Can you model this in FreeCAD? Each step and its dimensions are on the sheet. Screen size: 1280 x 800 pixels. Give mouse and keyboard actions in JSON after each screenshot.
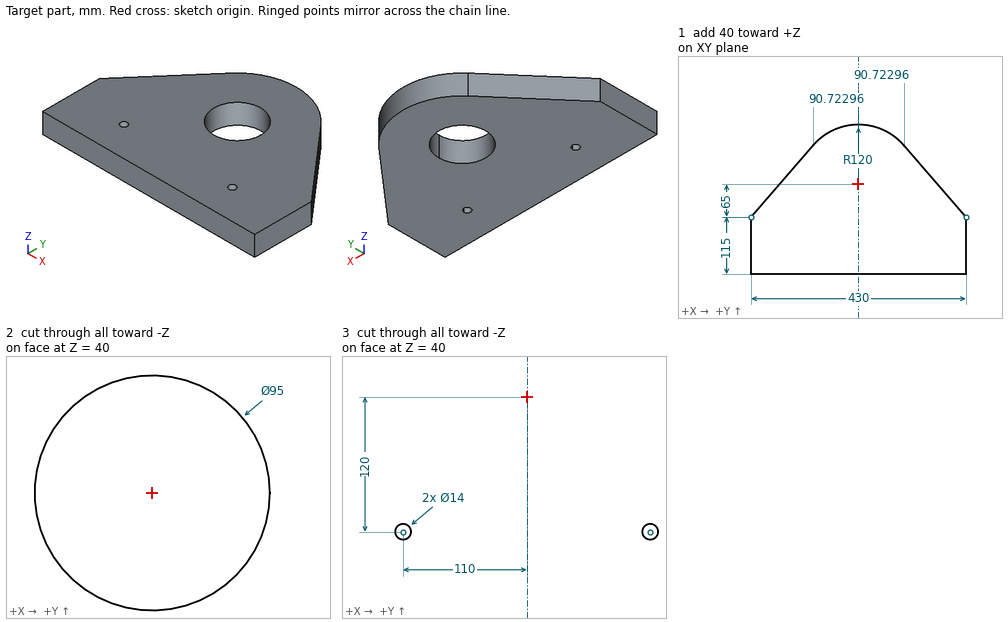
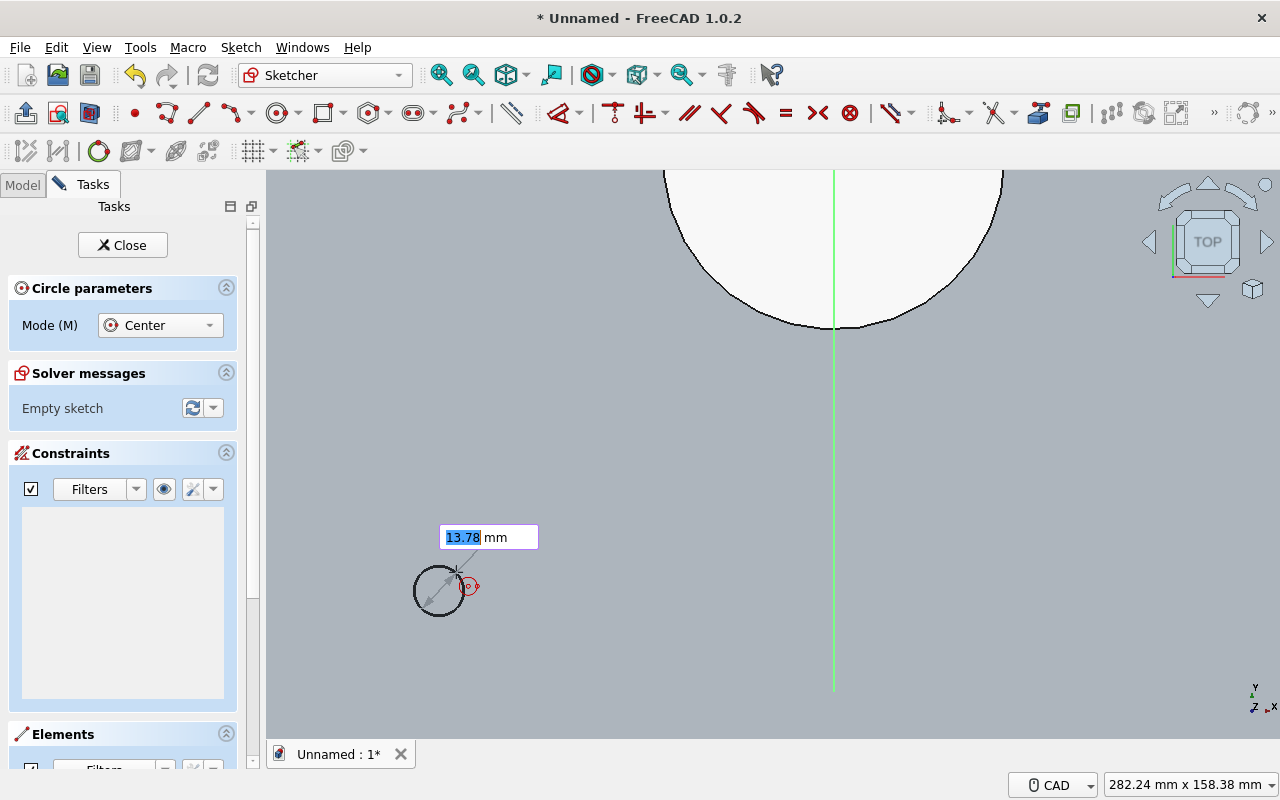
{"action": "type", "text": "14"}
{"action": "key", "text": "Return"}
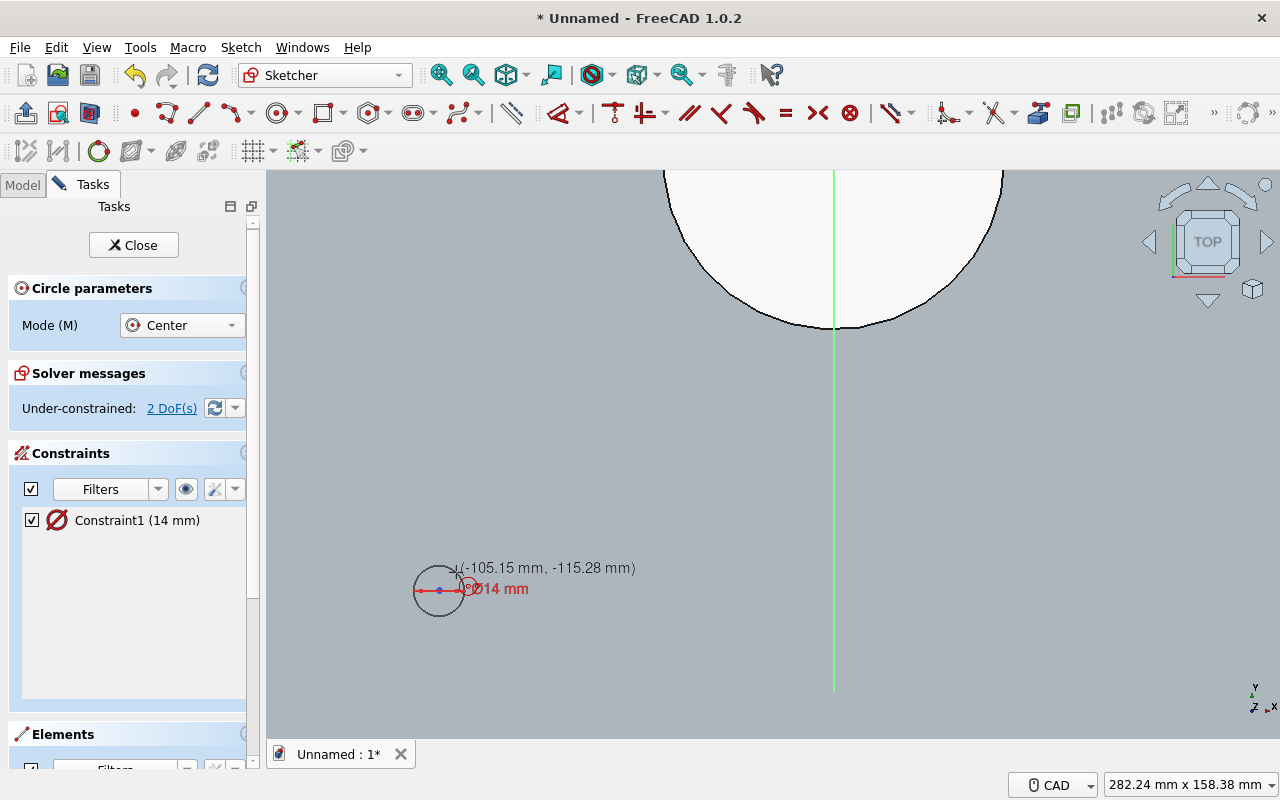
{"action": "scroll", "coordinate": [442, 592], "scroll_direction": "down", "scroll_amount": 2}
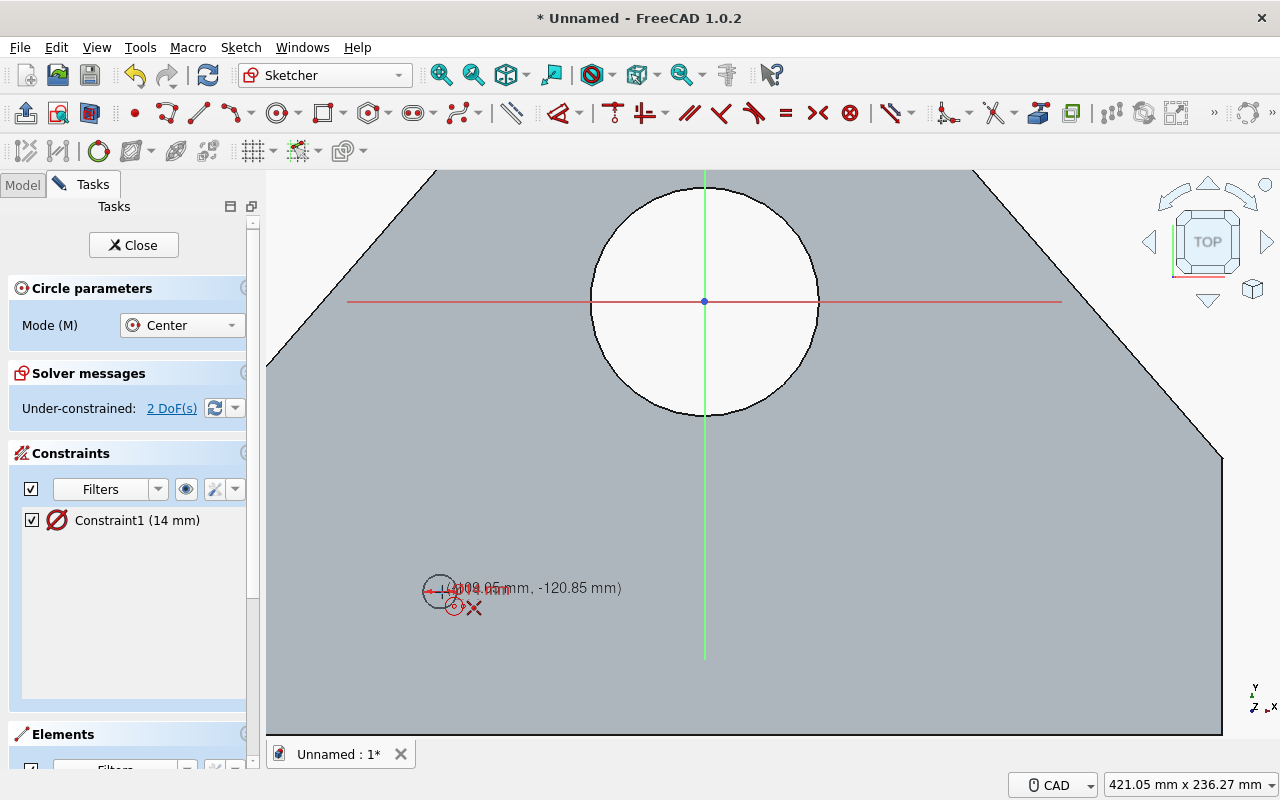
{"action": "scroll", "coordinate": [970, 591], "scroll_direction": "up", "scroll_amount": 2}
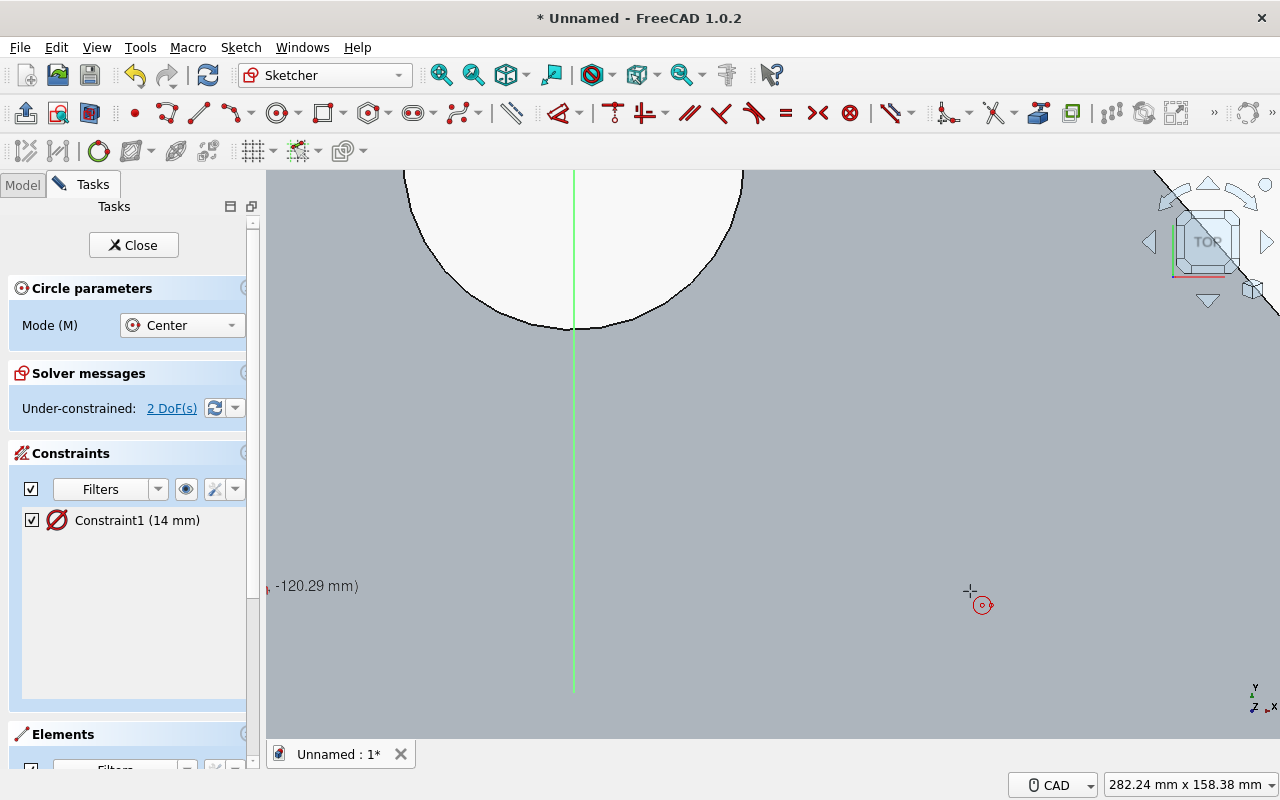
{"action": "left_click", "coordinate": [969, 590]}
{"action": "mouse_move", "coordinate": [987, 573]}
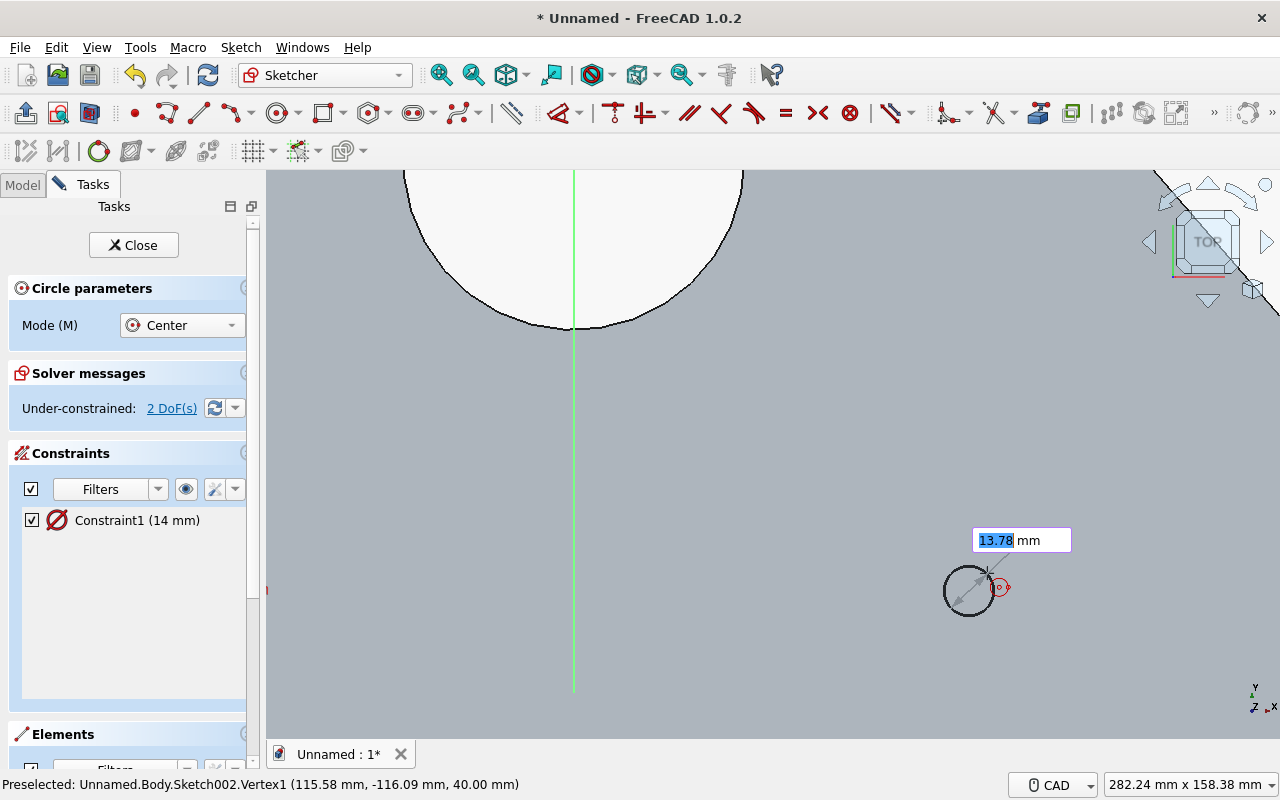
{"action": "type", "text": "14"}
{"action": "key", "text": "Return"}
{"action": "key", "text": "Escape"}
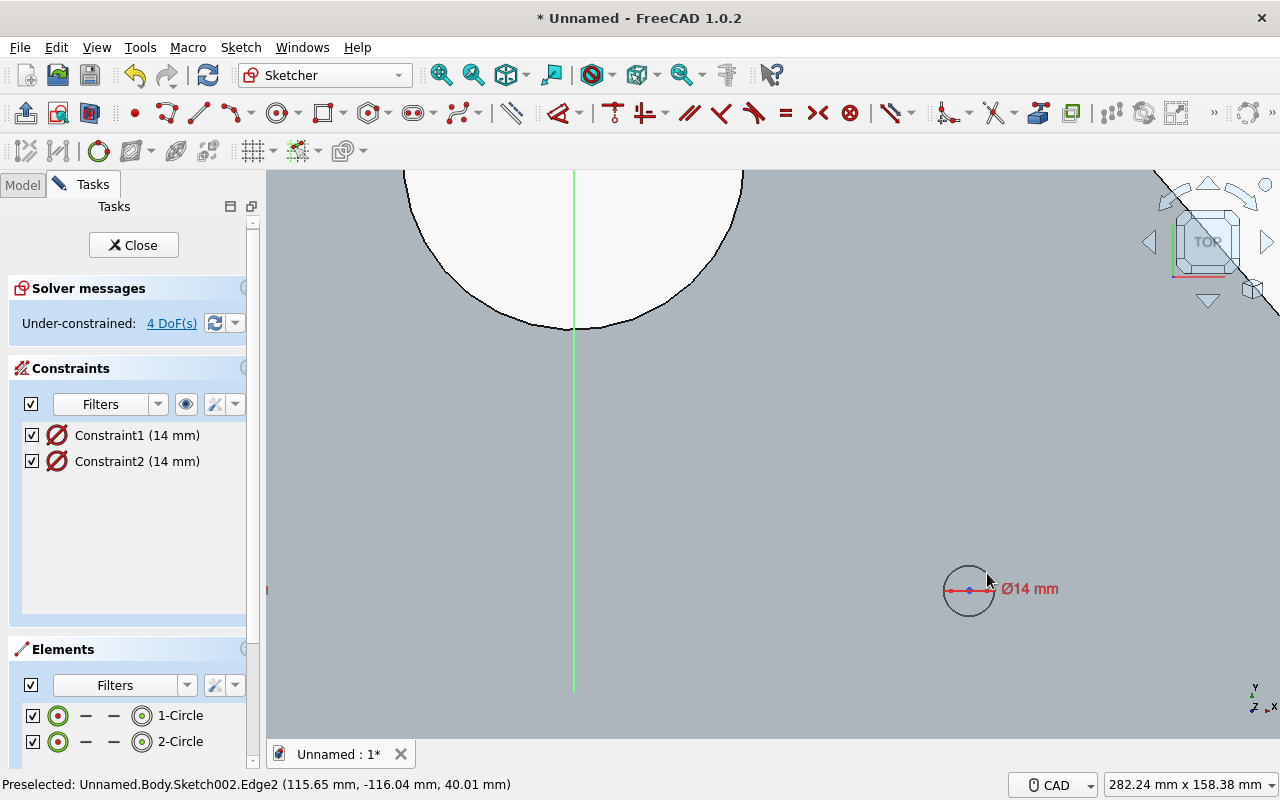
{"action": "scroll", "coordinate": [970, 591], "scroll_direction": "down", "scroll_amount": 2}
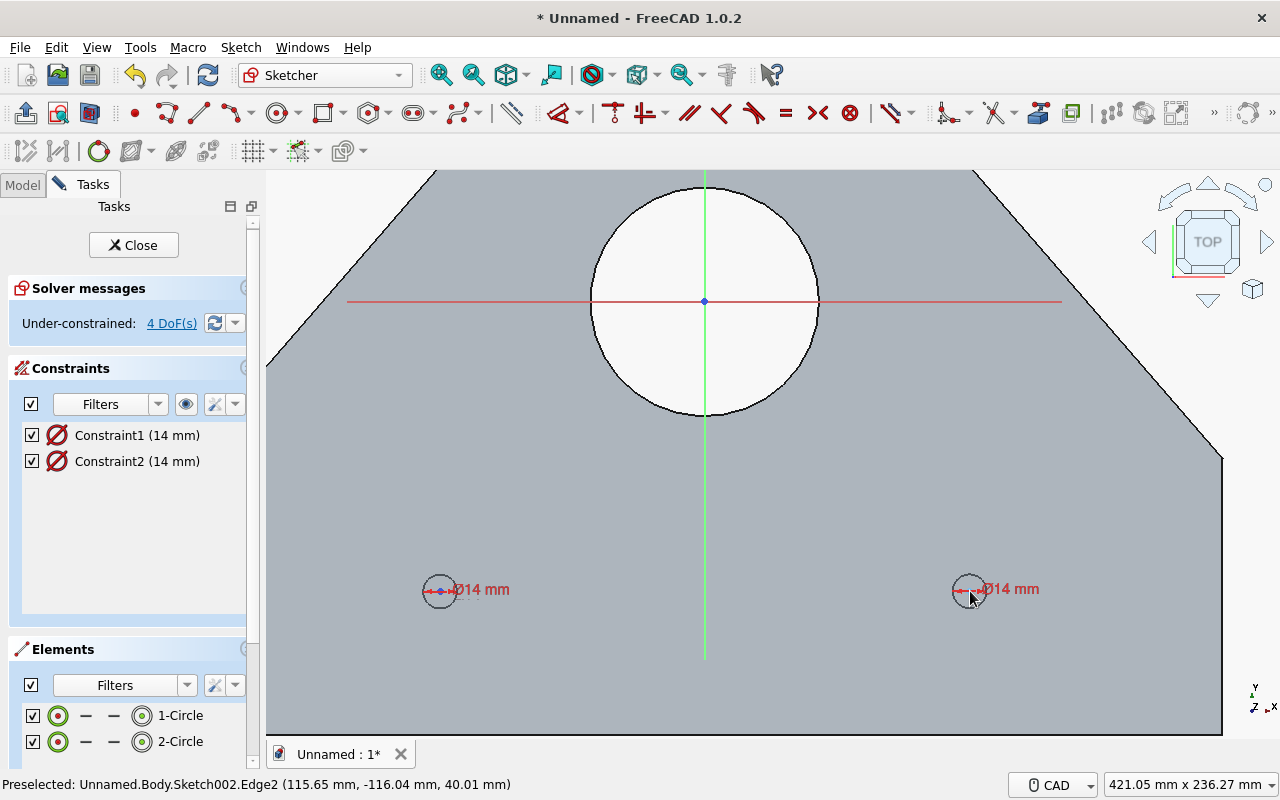
{"action": "left_click", "coordinate": [440, 592]}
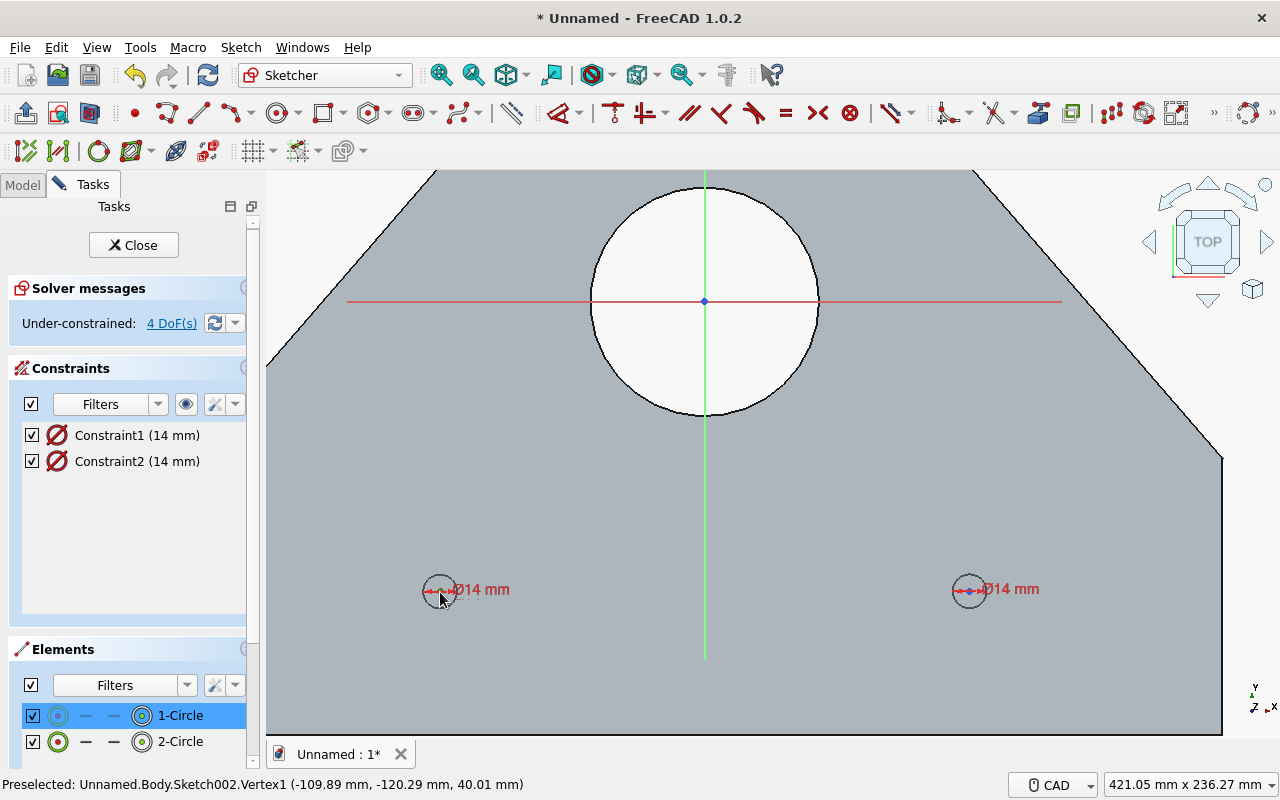
{"action": "left_click", "coordinate": [970, 591]}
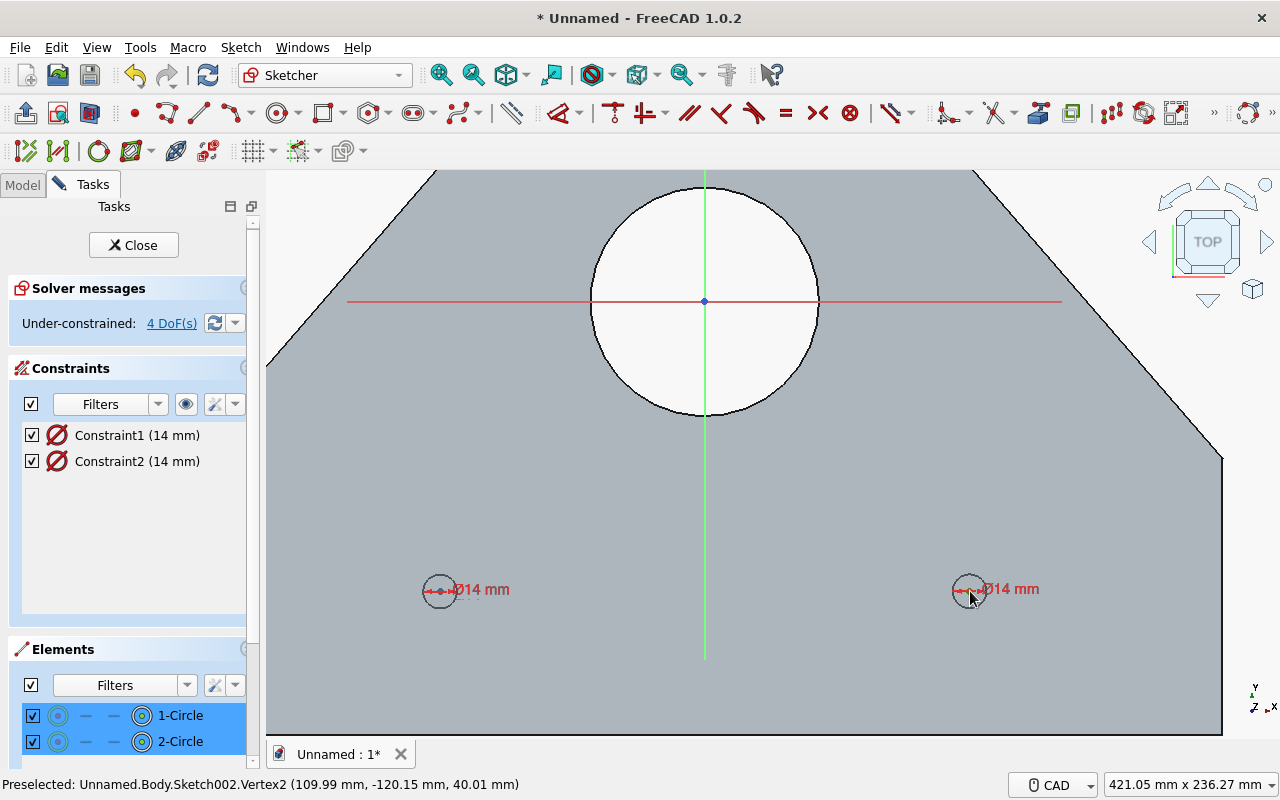
{"action": "left_click", "coordinate": [705, 638]}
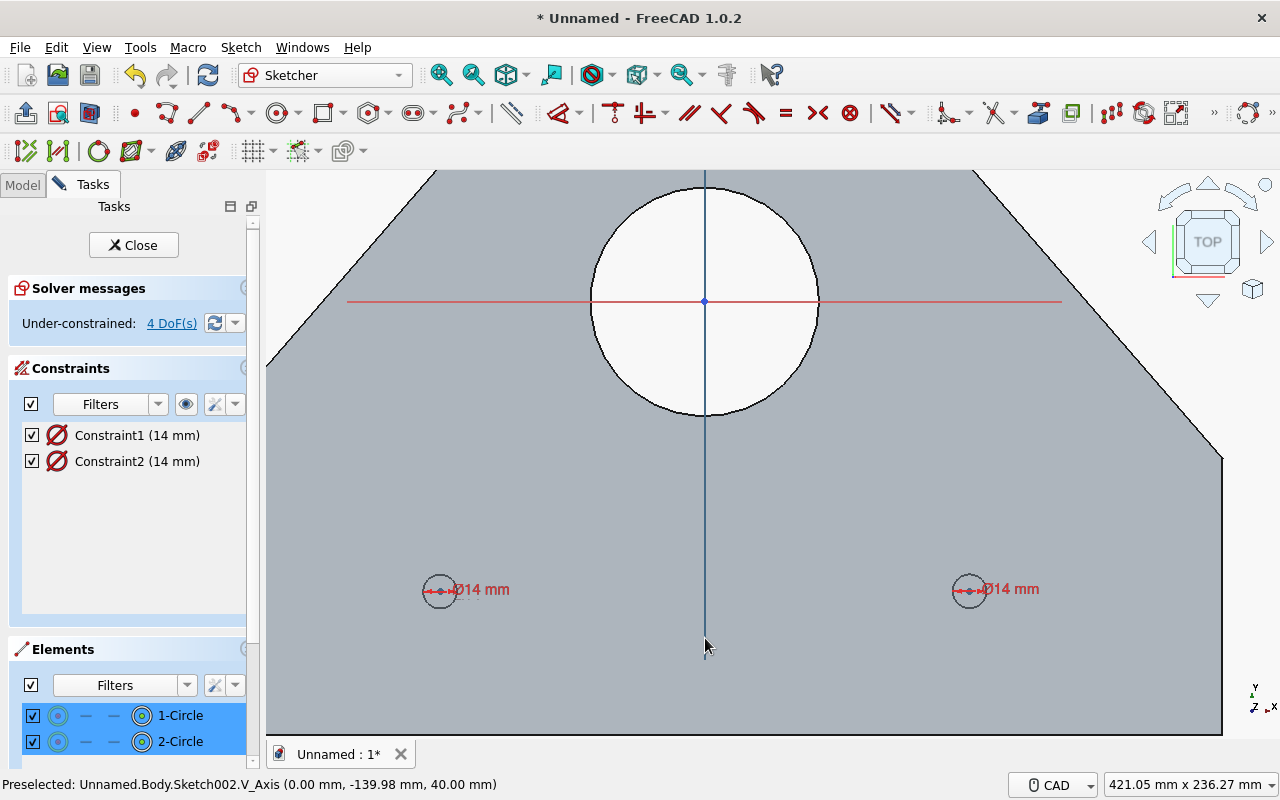
{"action": "left_click", "coordinate": [818, 114]}